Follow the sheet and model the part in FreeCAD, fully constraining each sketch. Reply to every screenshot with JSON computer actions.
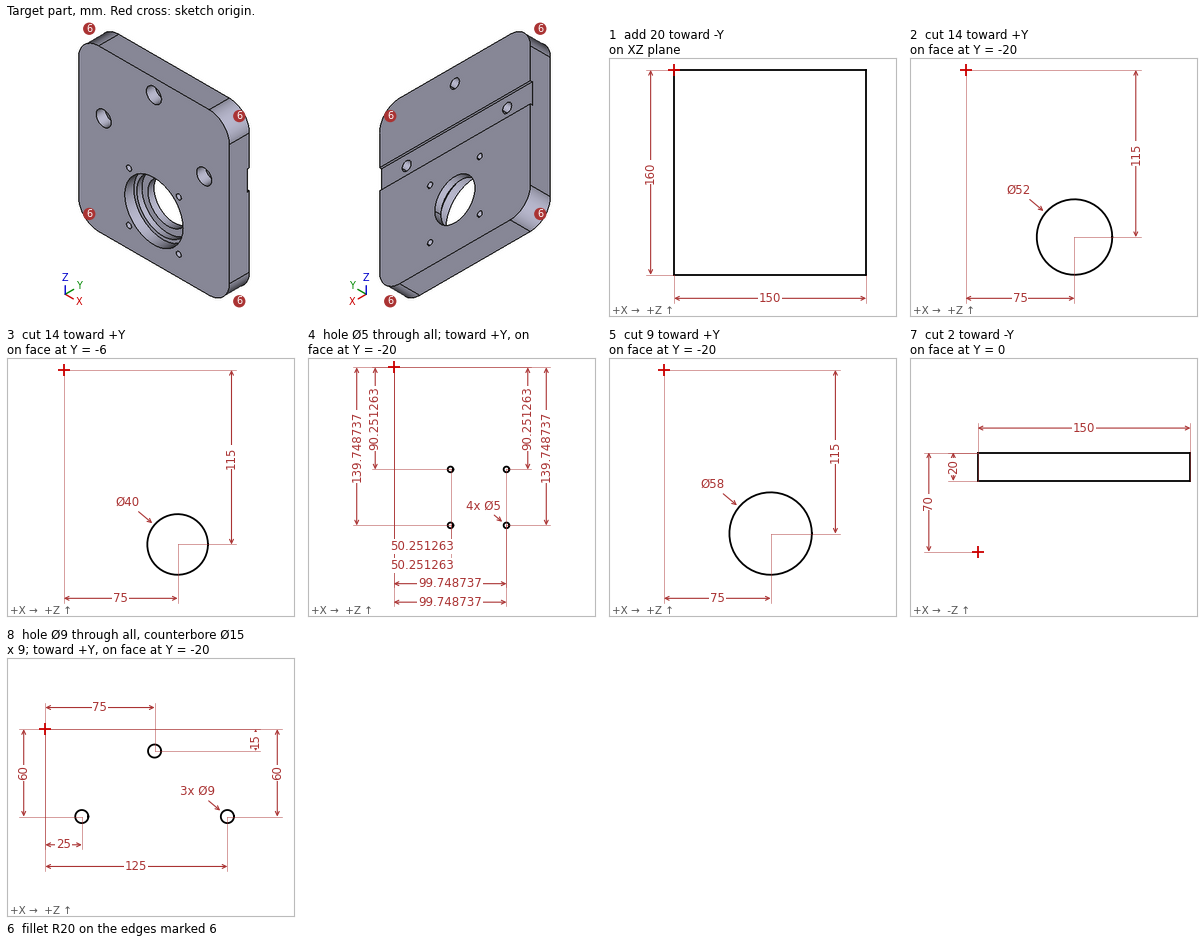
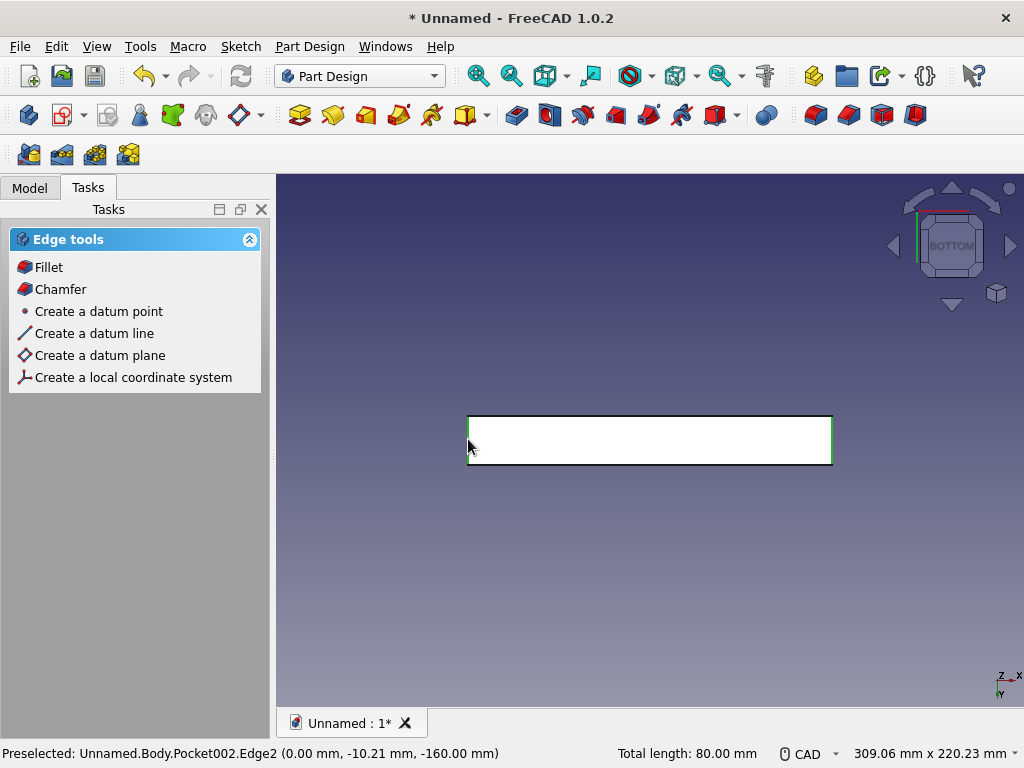
{"action": "left_click", "coordinate": [816, 116]}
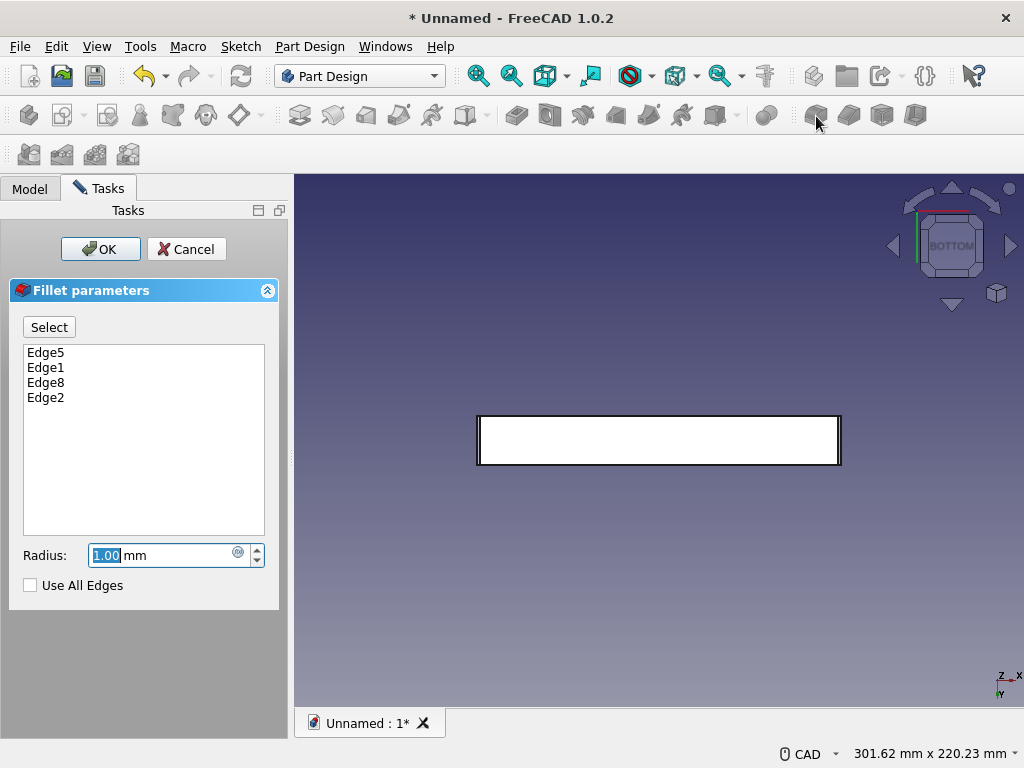
{"action": "type", "text": "20"}
{"action": "key", "text": "Tab"}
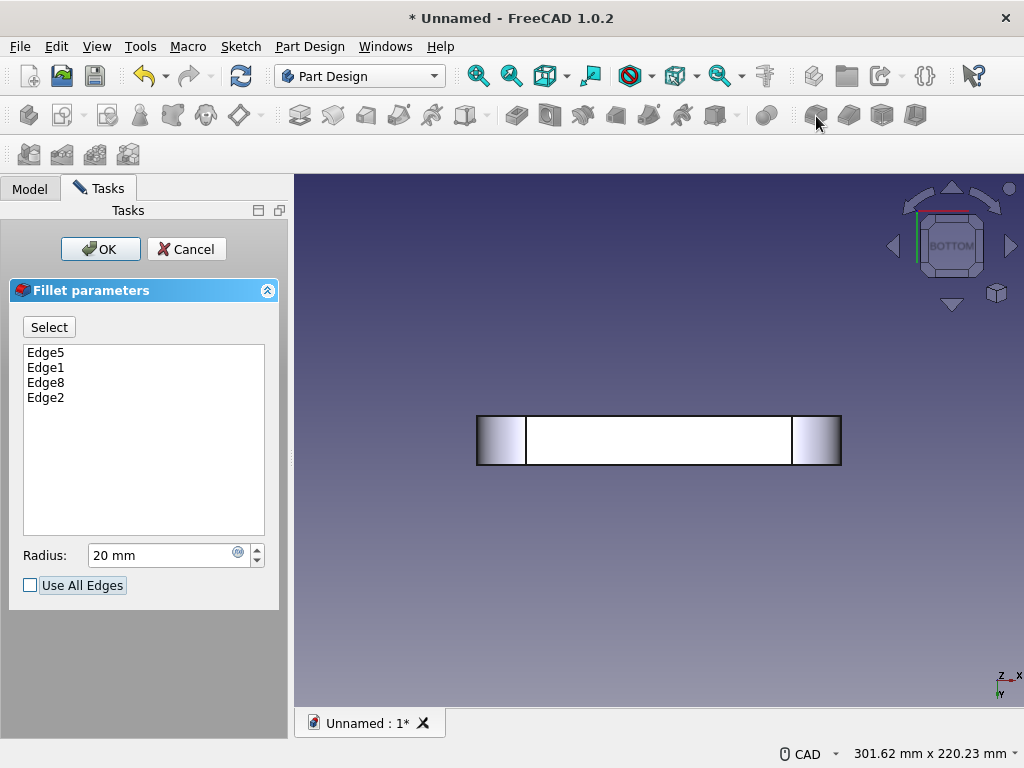
{"action": "left_click", "coordinate": [101, 249]}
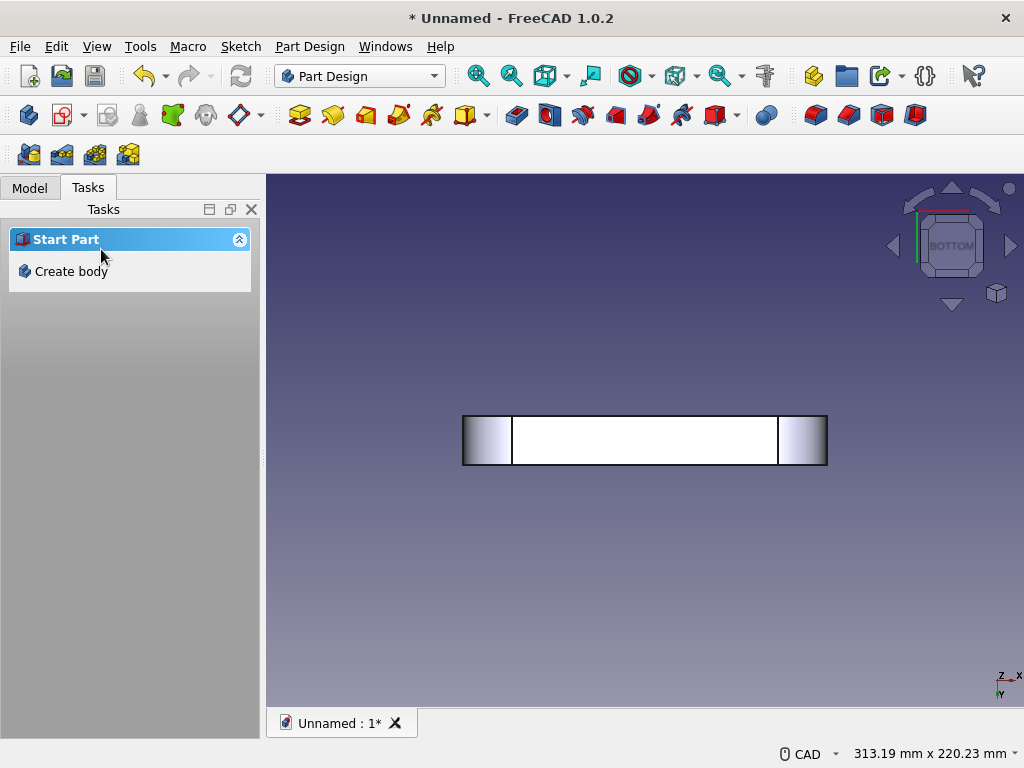
{"action": "key", "text": "4"}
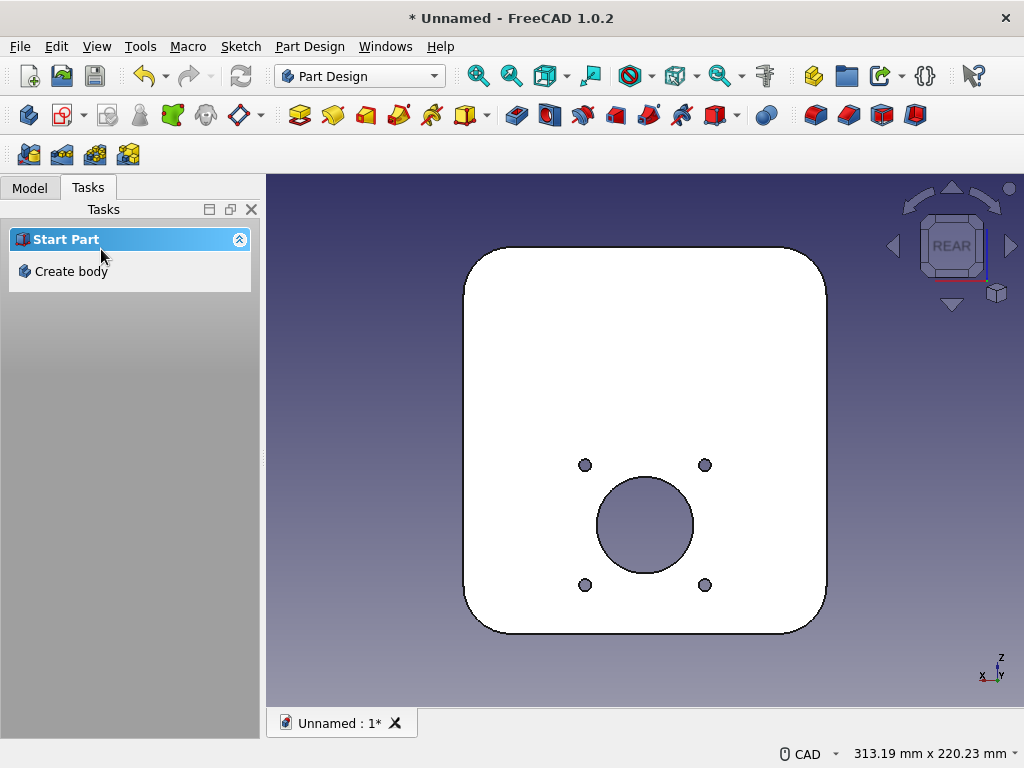
{"action": "left_click", "coordinate": [645, 384]}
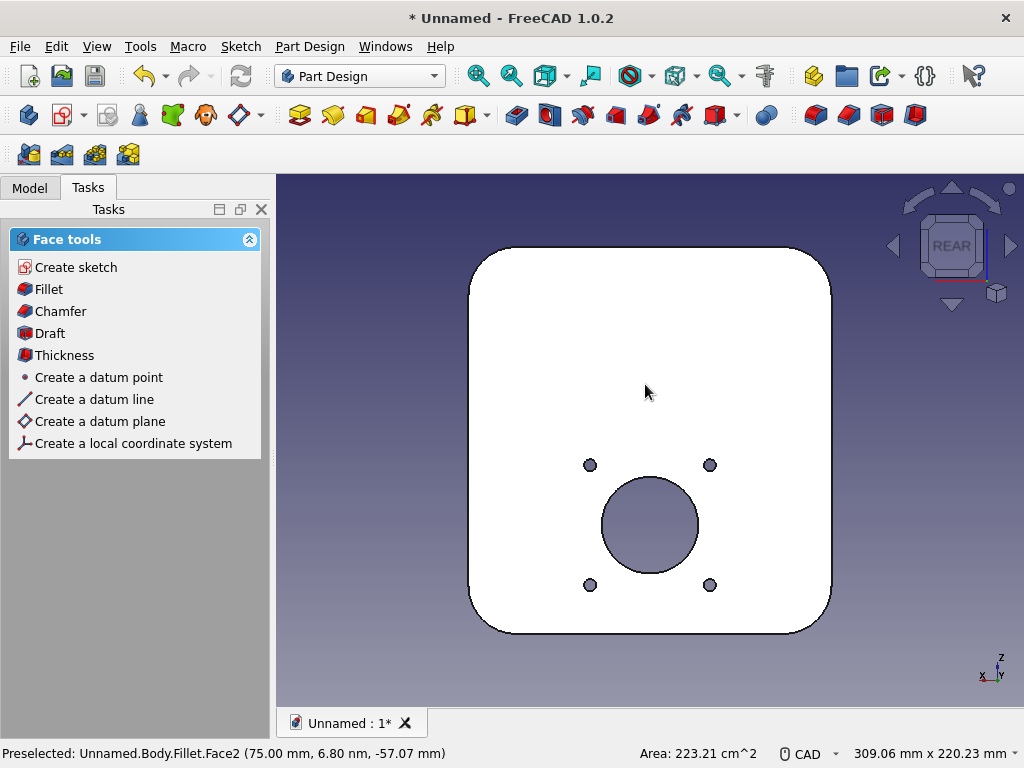
{"action": "left_click", "coordinate": [62, 116]}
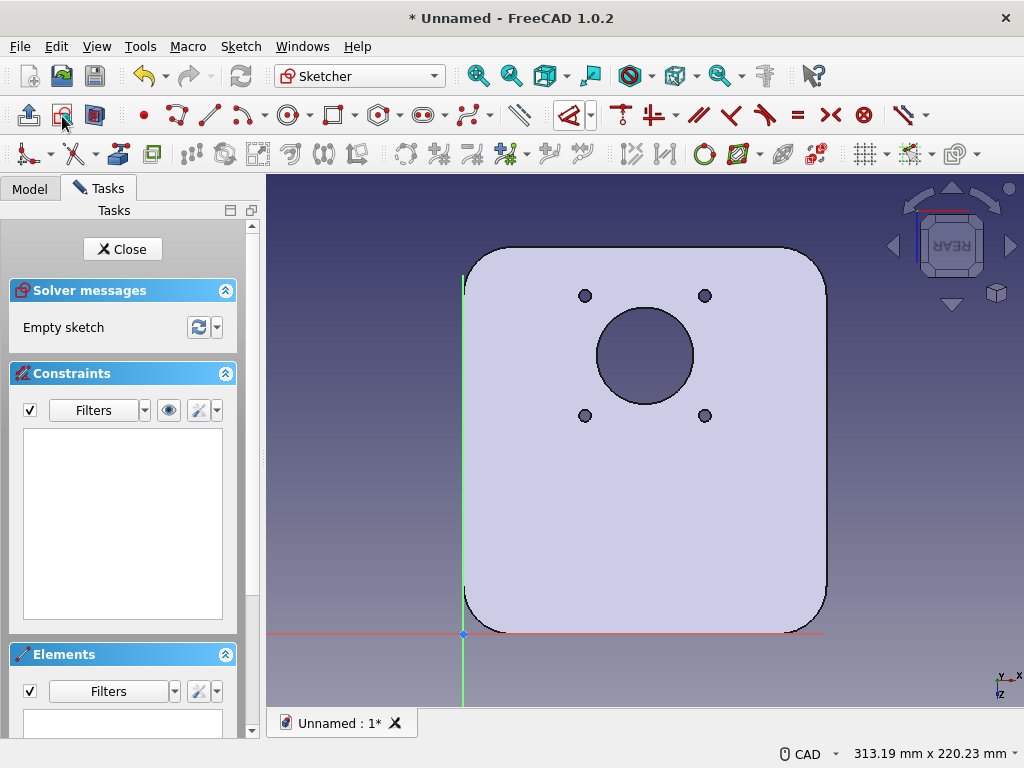
{"action": "left_click", "coordinate": [332, 116]}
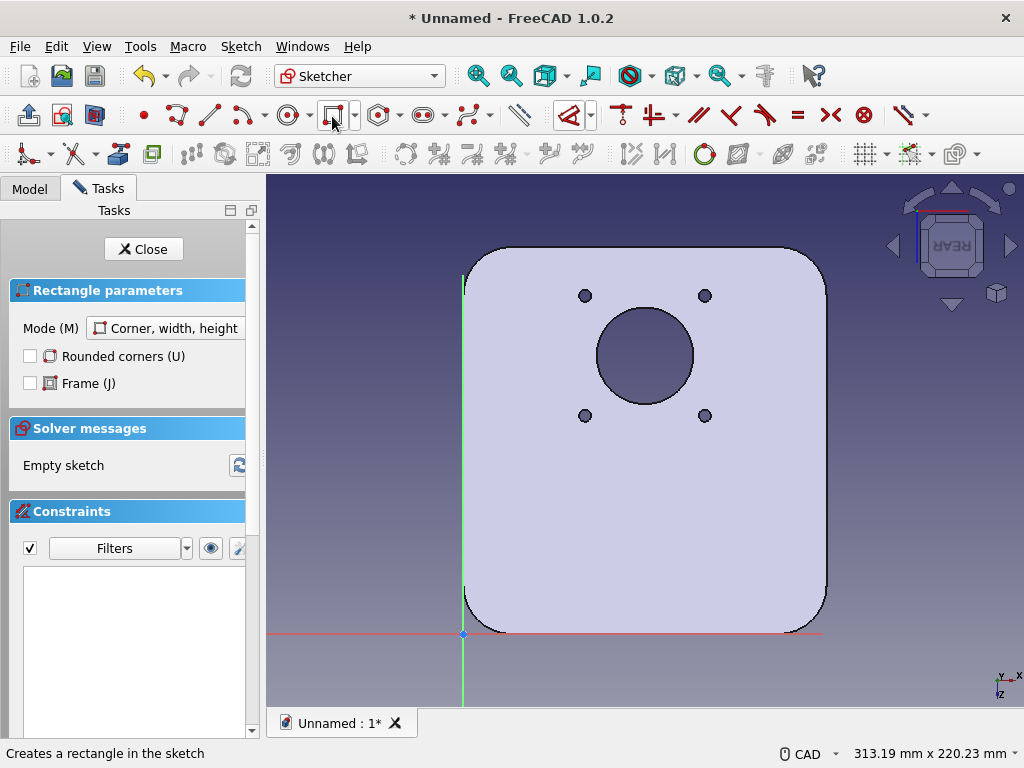
{"action": "left_click", "coordinate": [463, 465]}
{"action": "left_click", "coordinate": [827, 513]}
{"action": "key", "text": "Escape"}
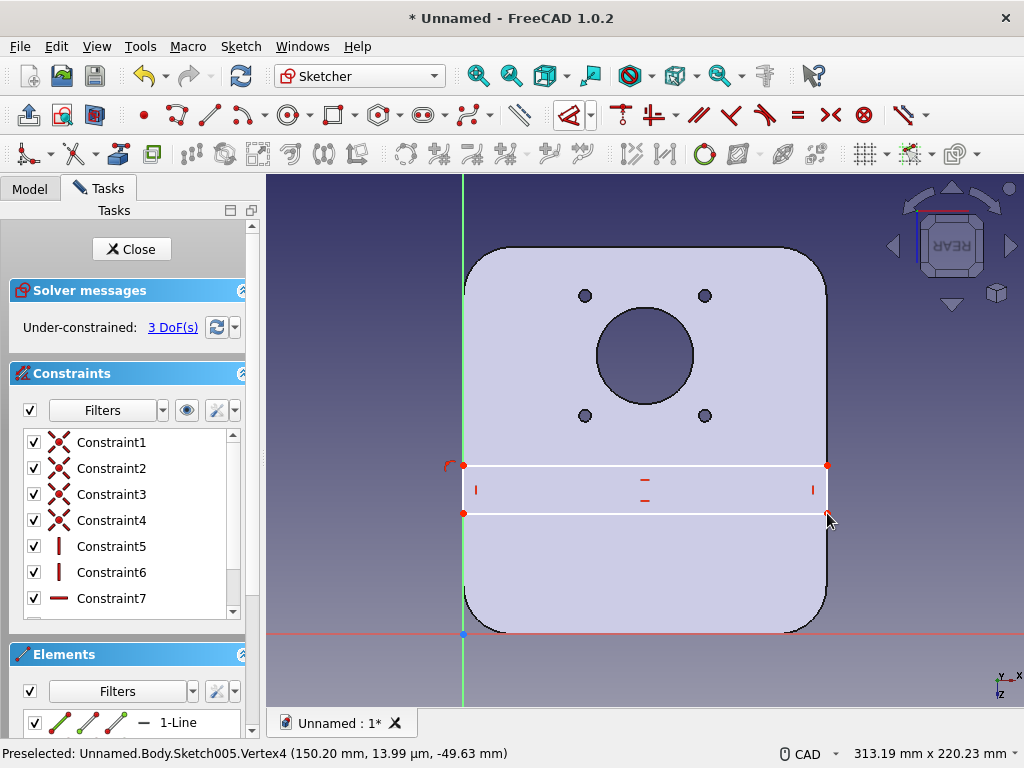
{"action": "left_click", "coordinate": [463, 480]}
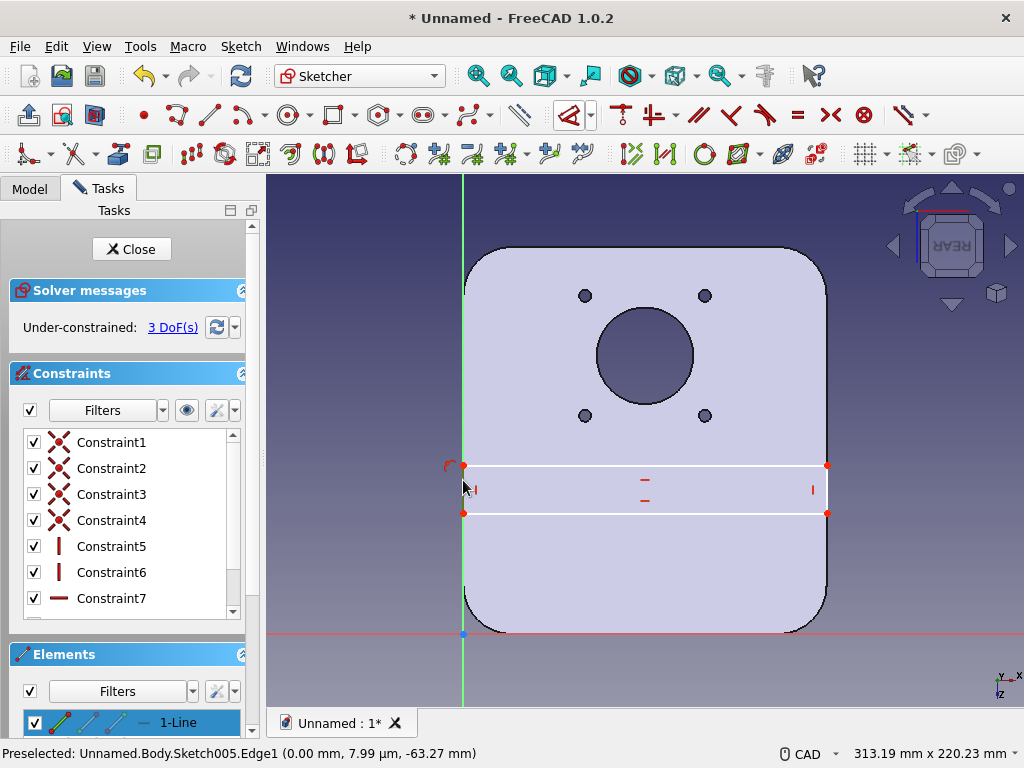
{"action": "left_click", "coordinate": [590, 116]}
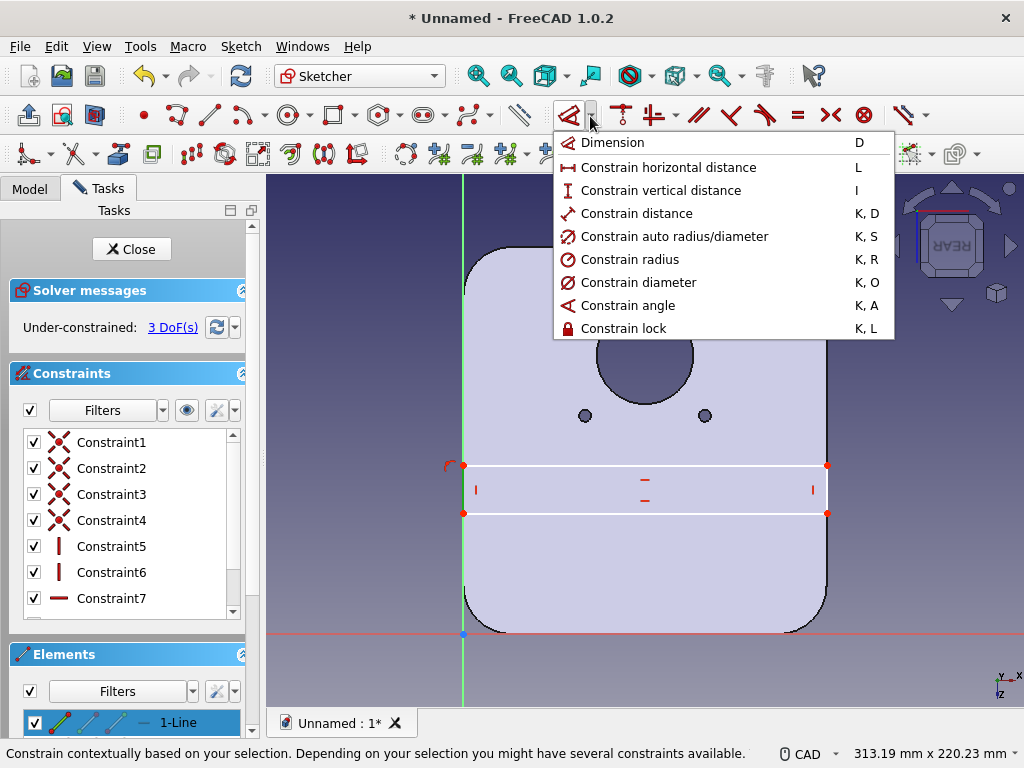
{"action": "left_click", "coordinate": [724, 190]}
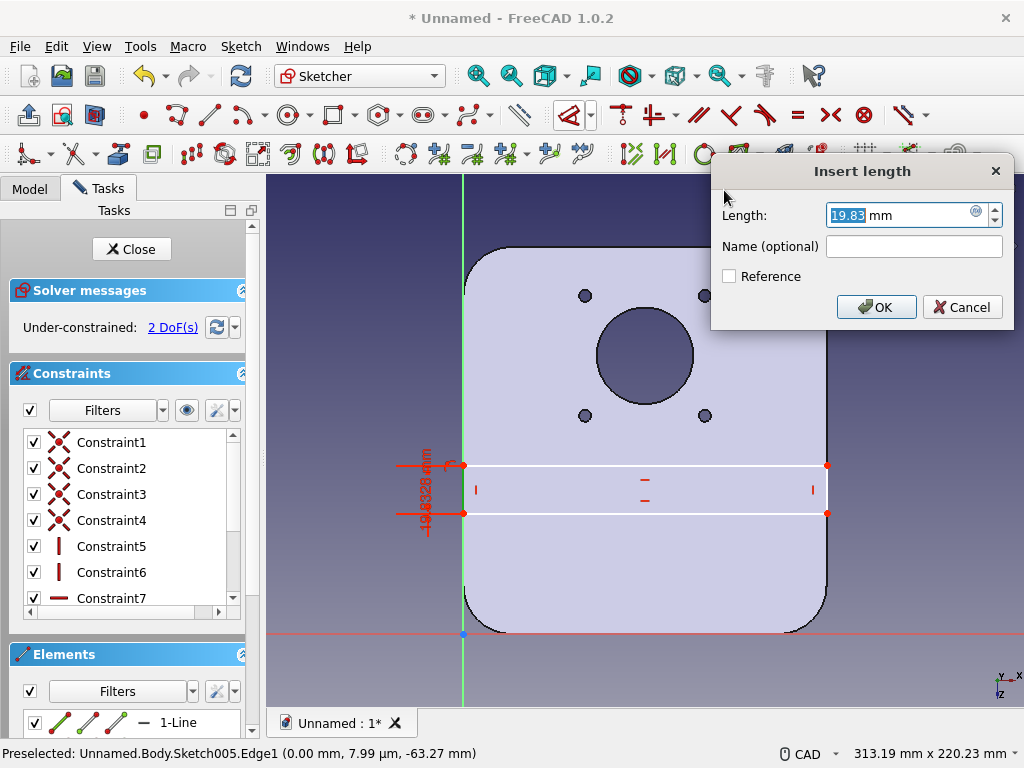
{"action": "type", "text": "20"}
{"action": "key", "text": "Return"}